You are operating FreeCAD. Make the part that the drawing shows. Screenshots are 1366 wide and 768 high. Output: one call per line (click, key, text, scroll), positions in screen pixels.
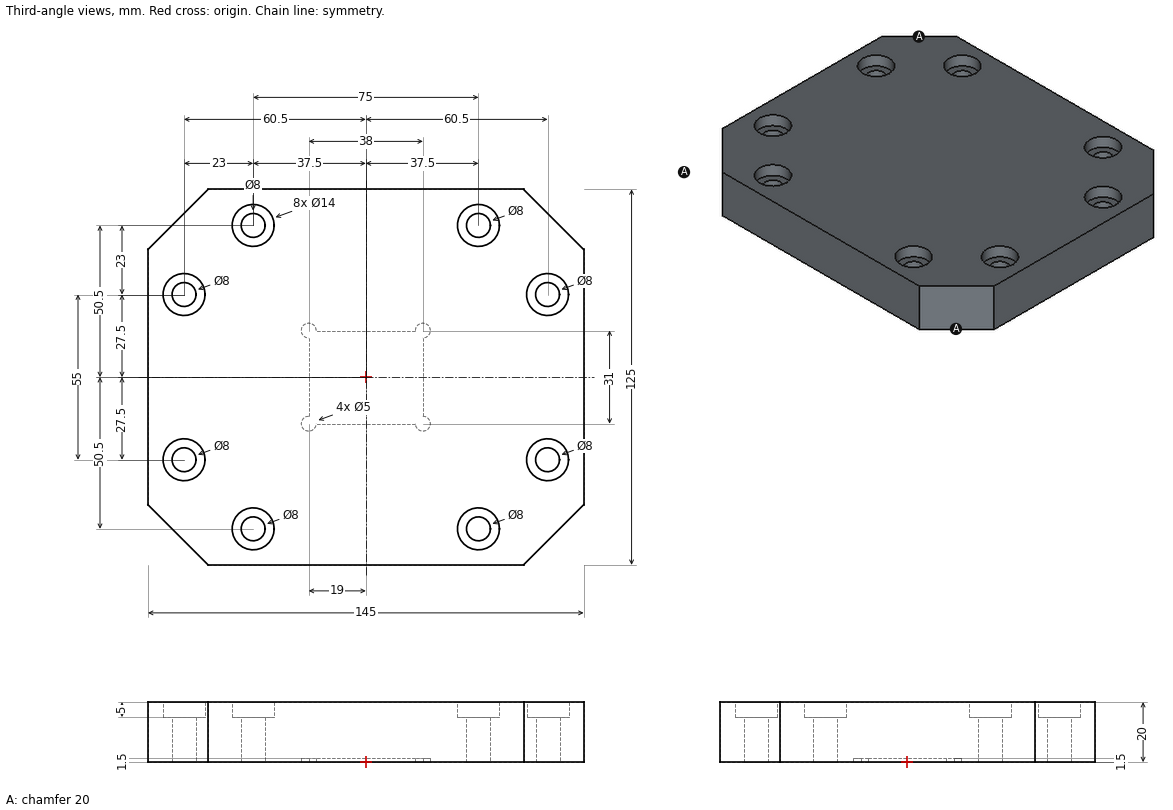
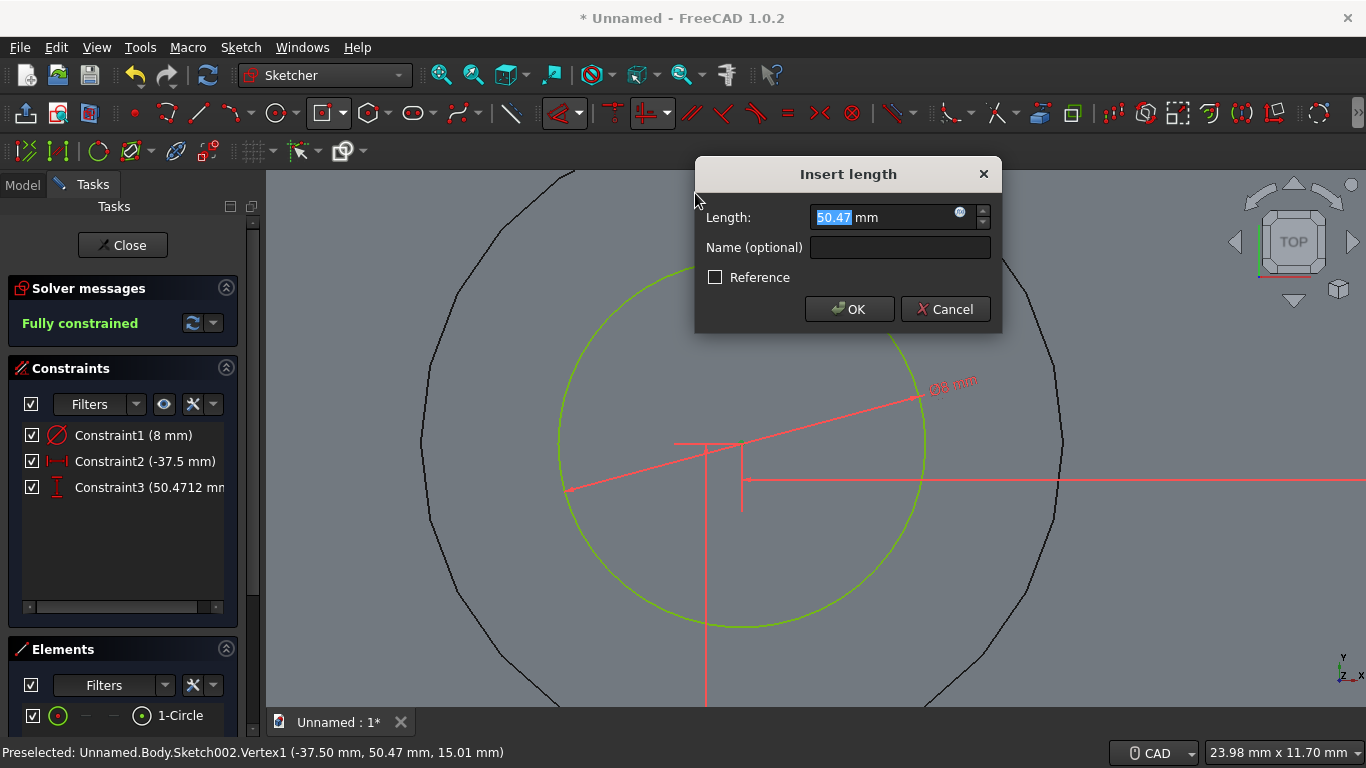
text(50.5)
key(Return)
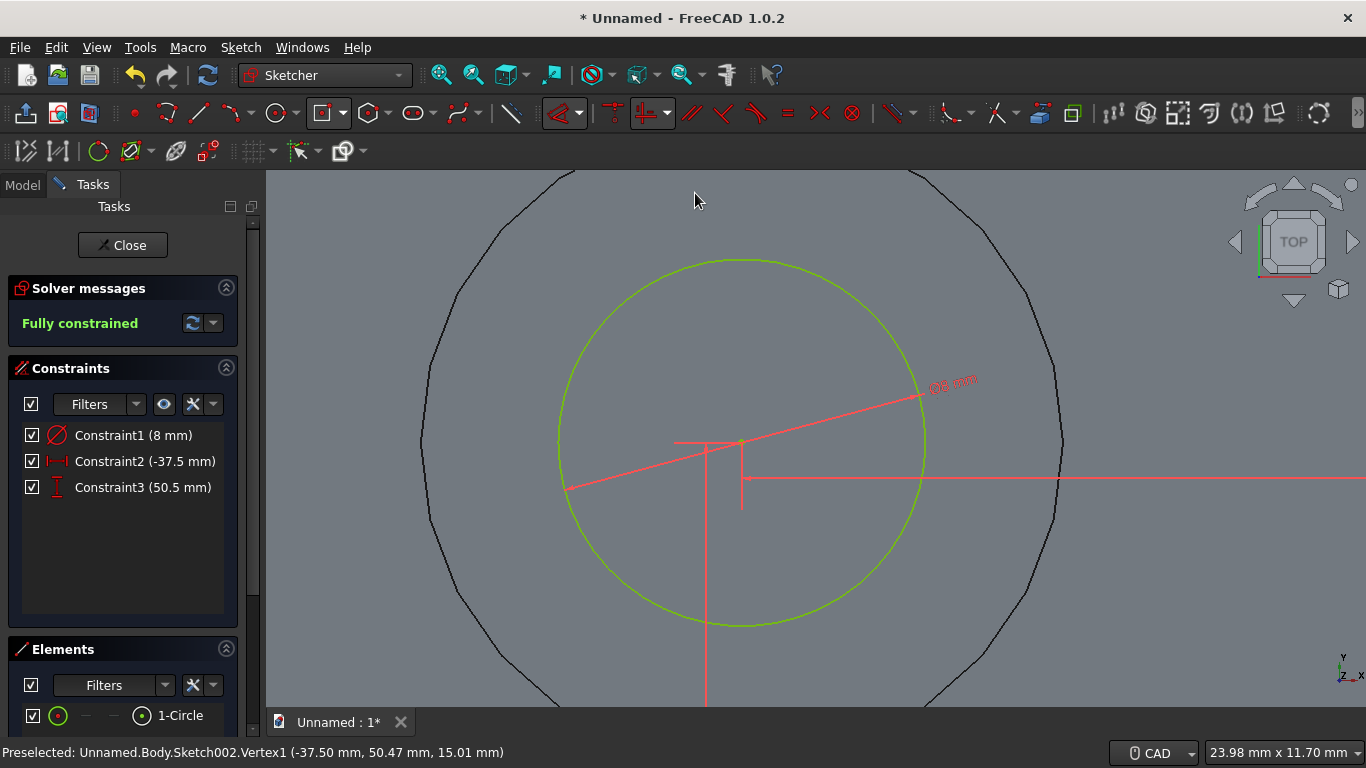
click(123, 245)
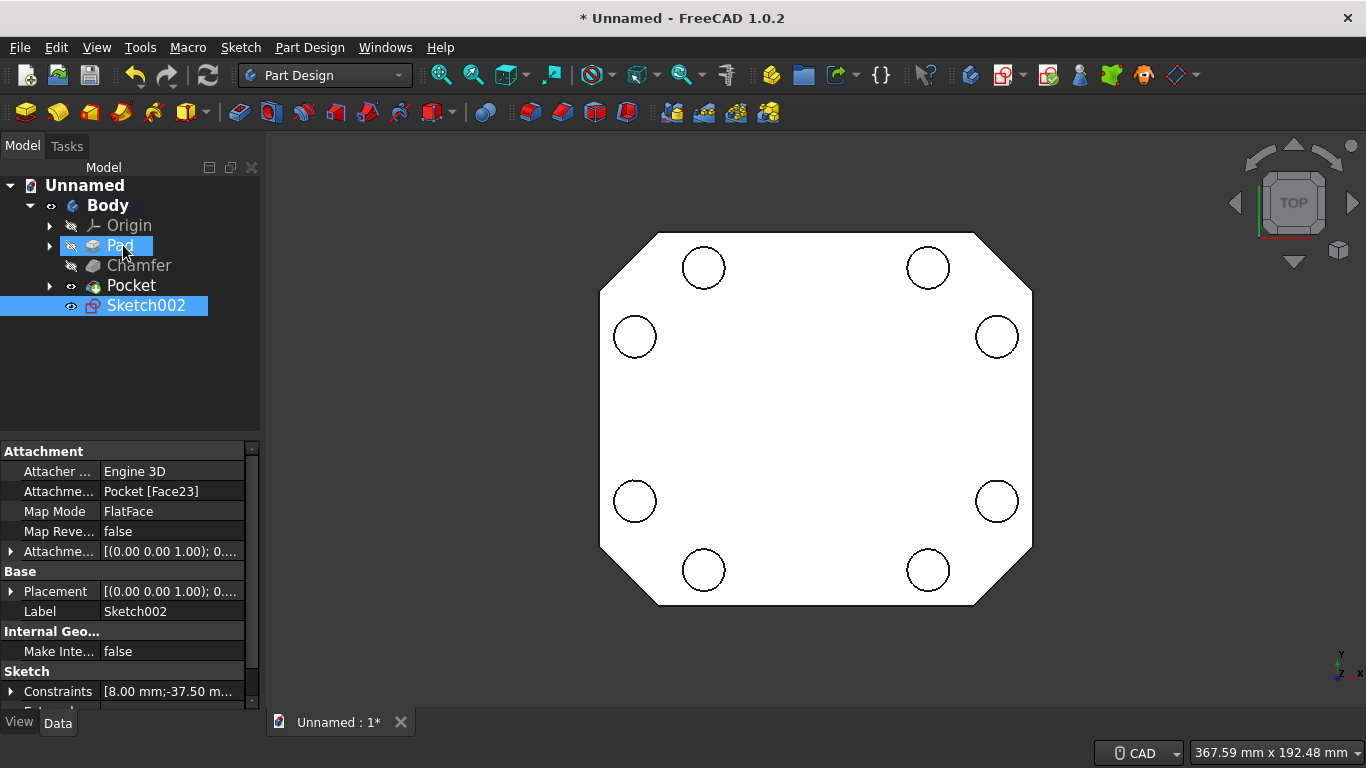
click(240, 112)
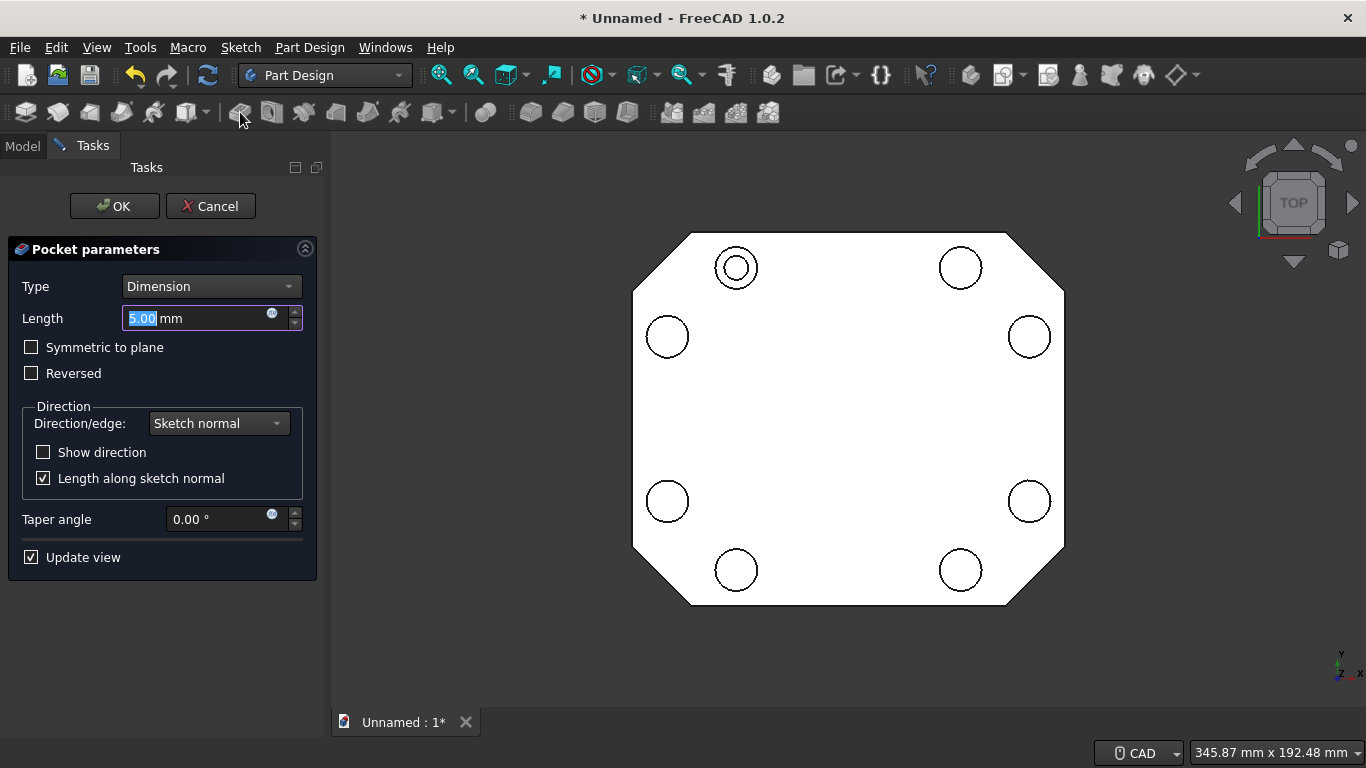
click(212, 286)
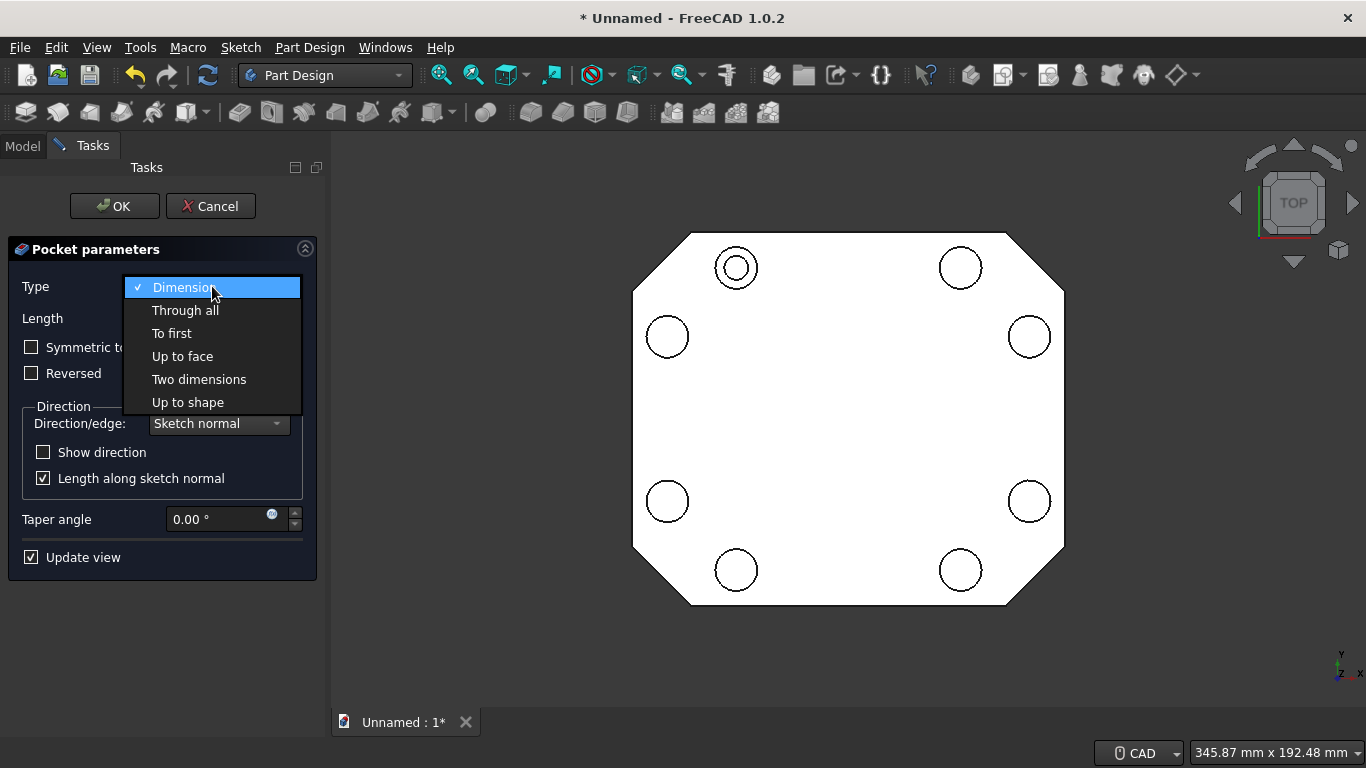
click(212, 334)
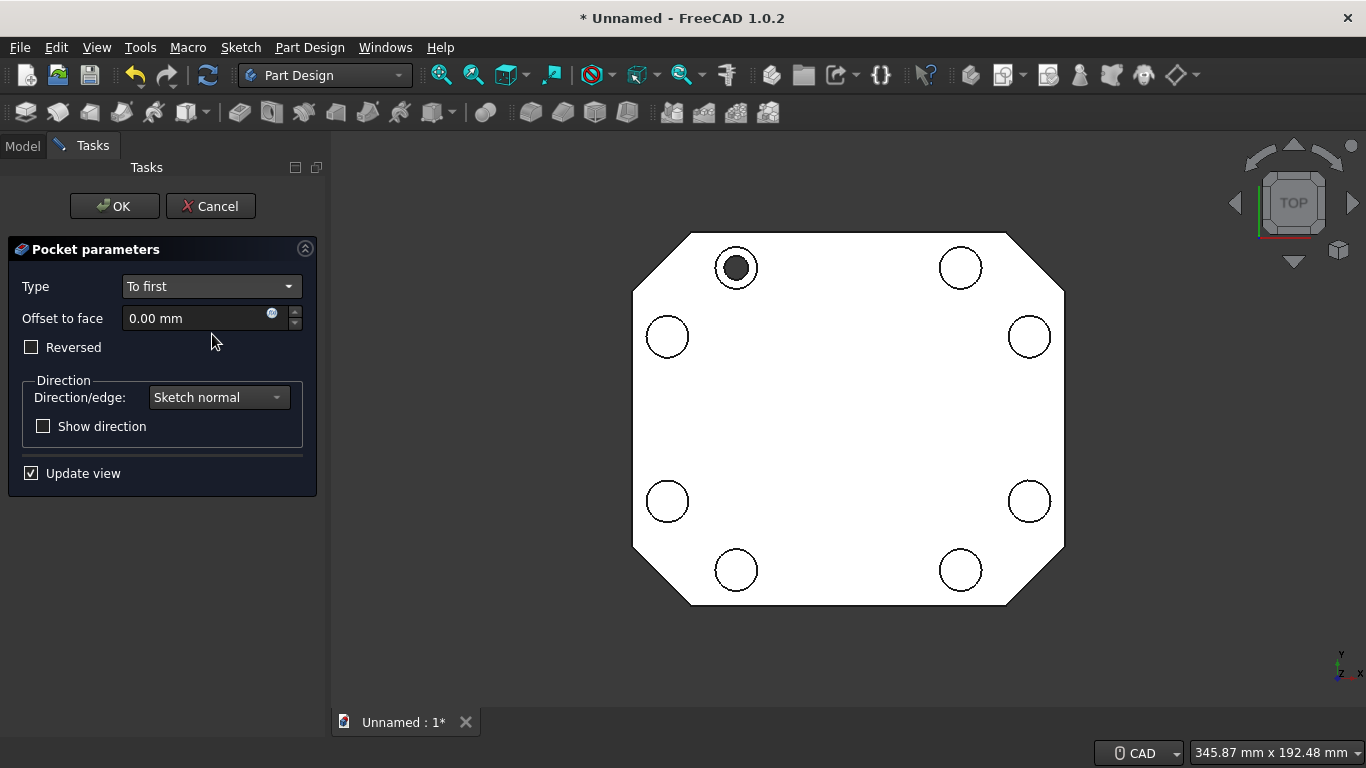
click(115, 206)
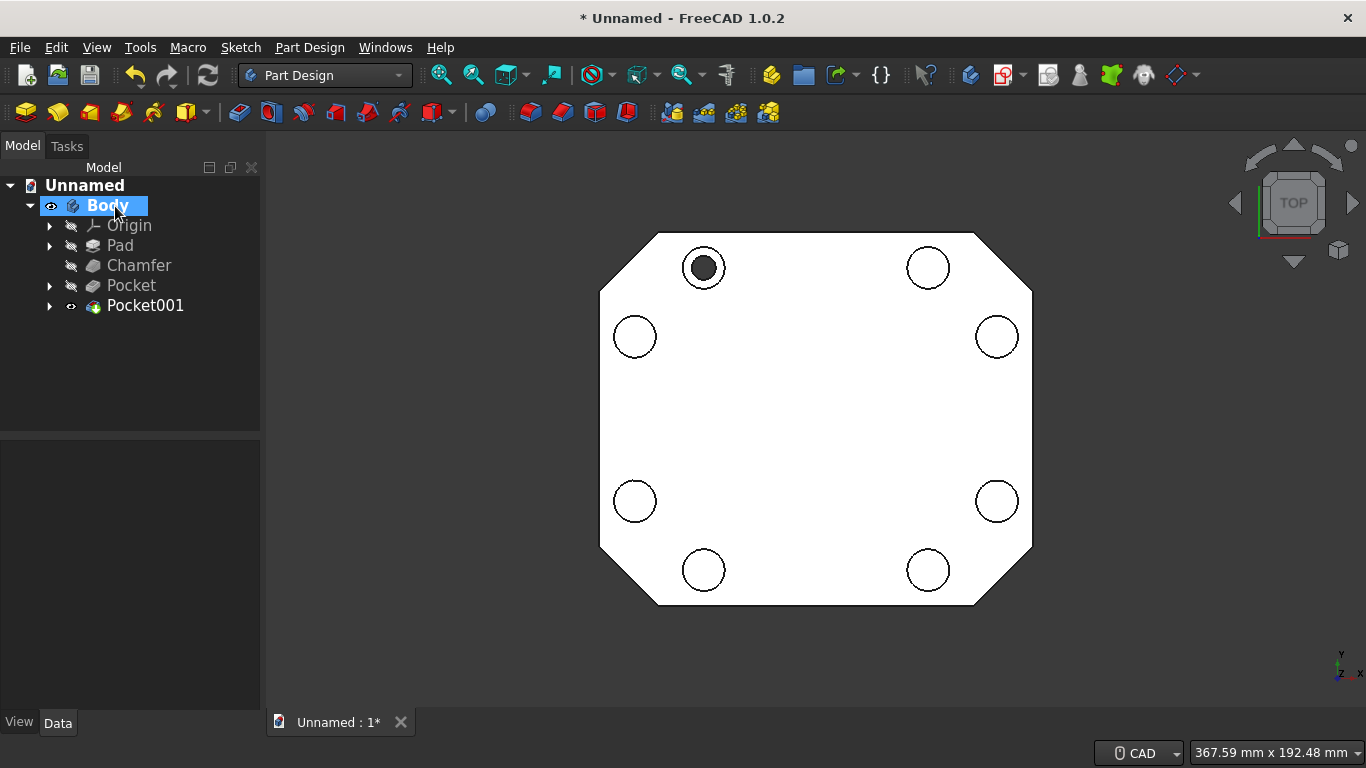
click(635, 336)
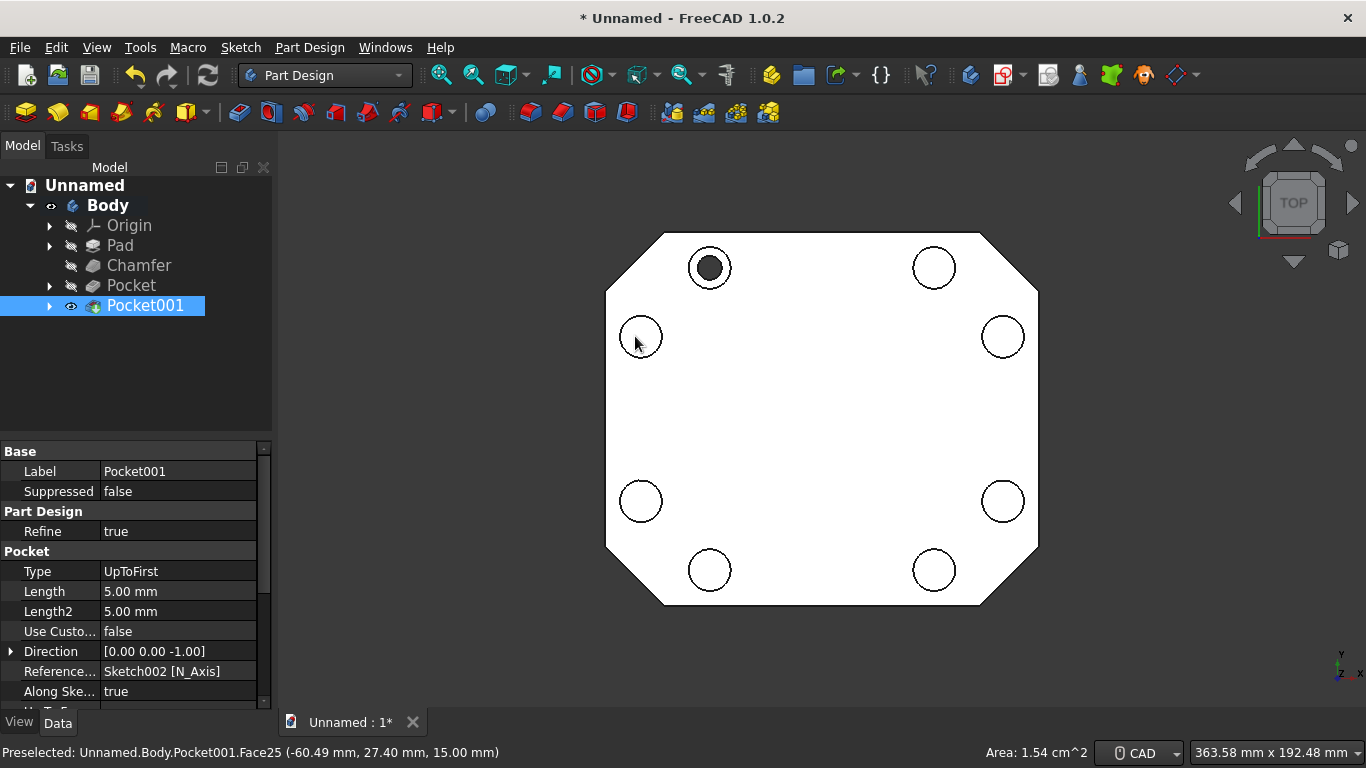
click(1004, 76)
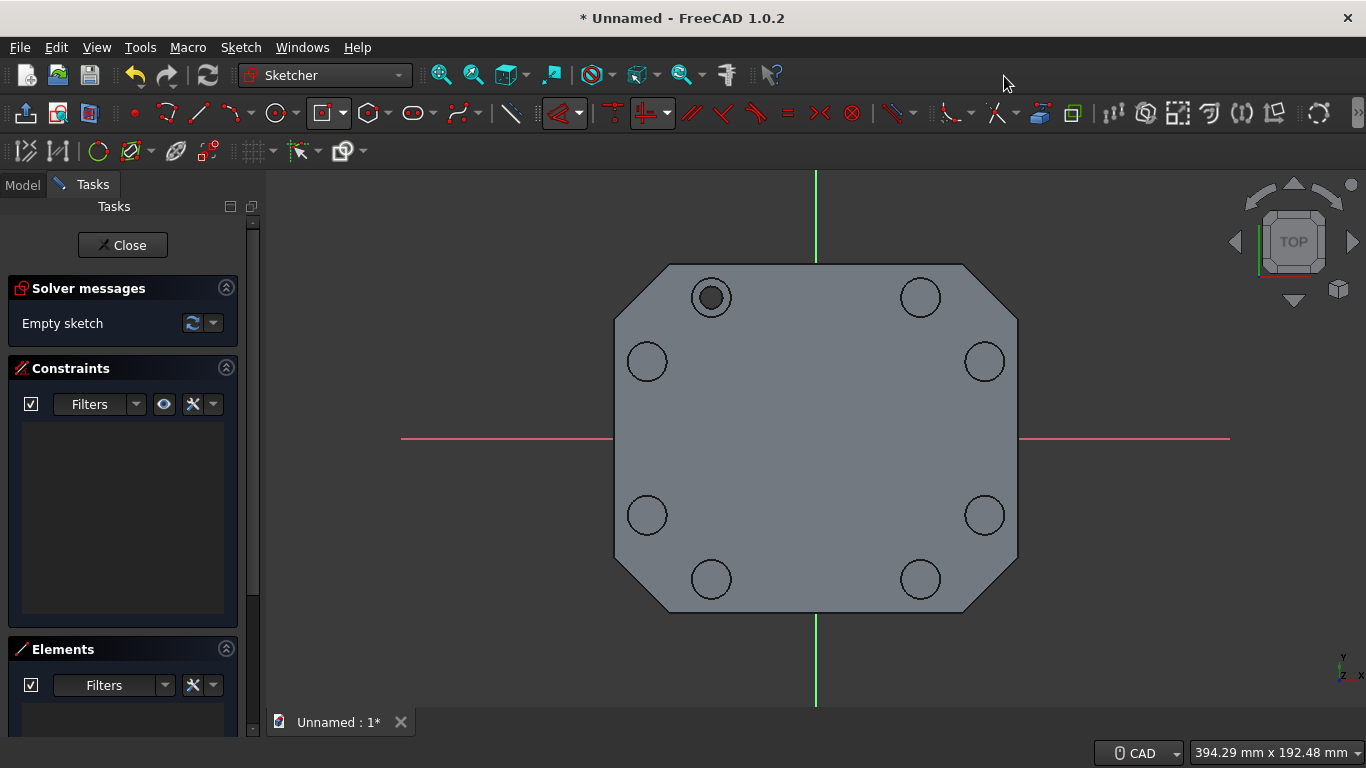
key(q)
key(s)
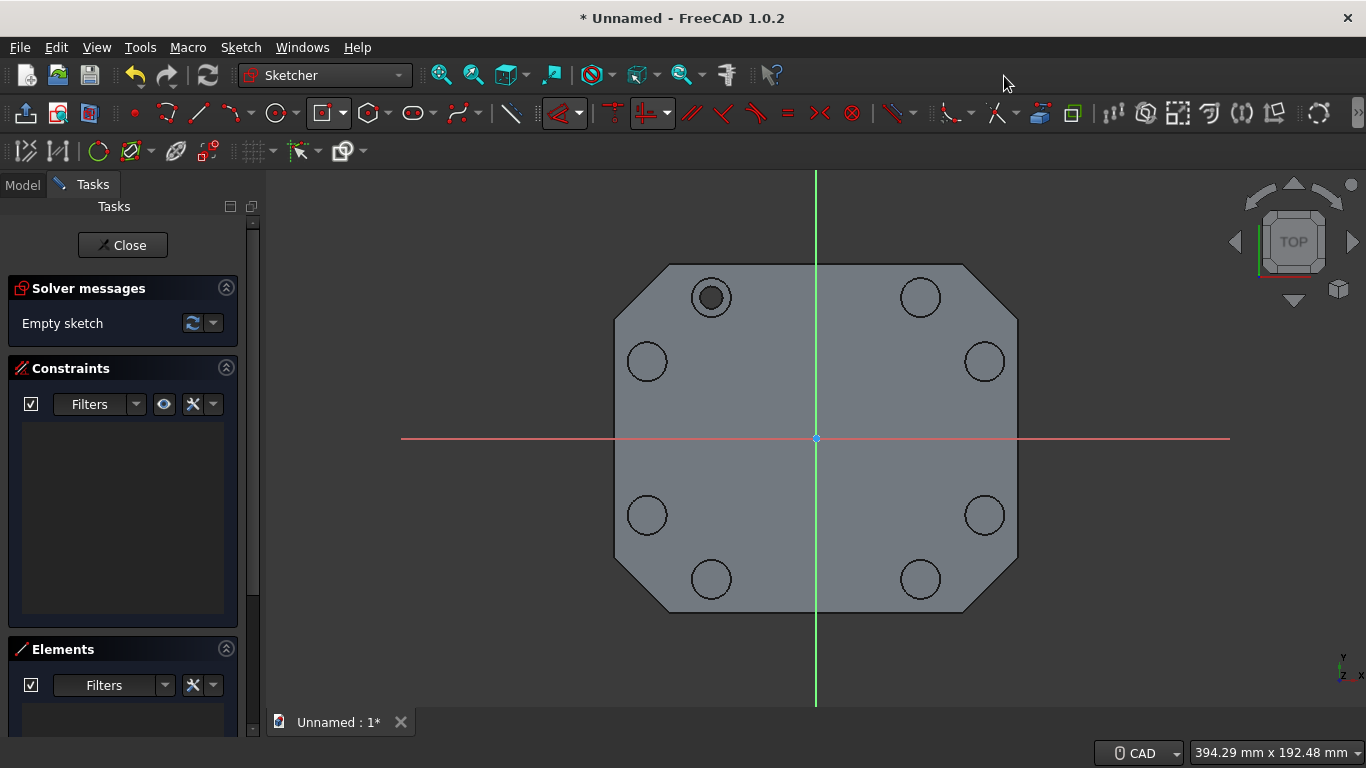
scroll(641, 357, up, 14)